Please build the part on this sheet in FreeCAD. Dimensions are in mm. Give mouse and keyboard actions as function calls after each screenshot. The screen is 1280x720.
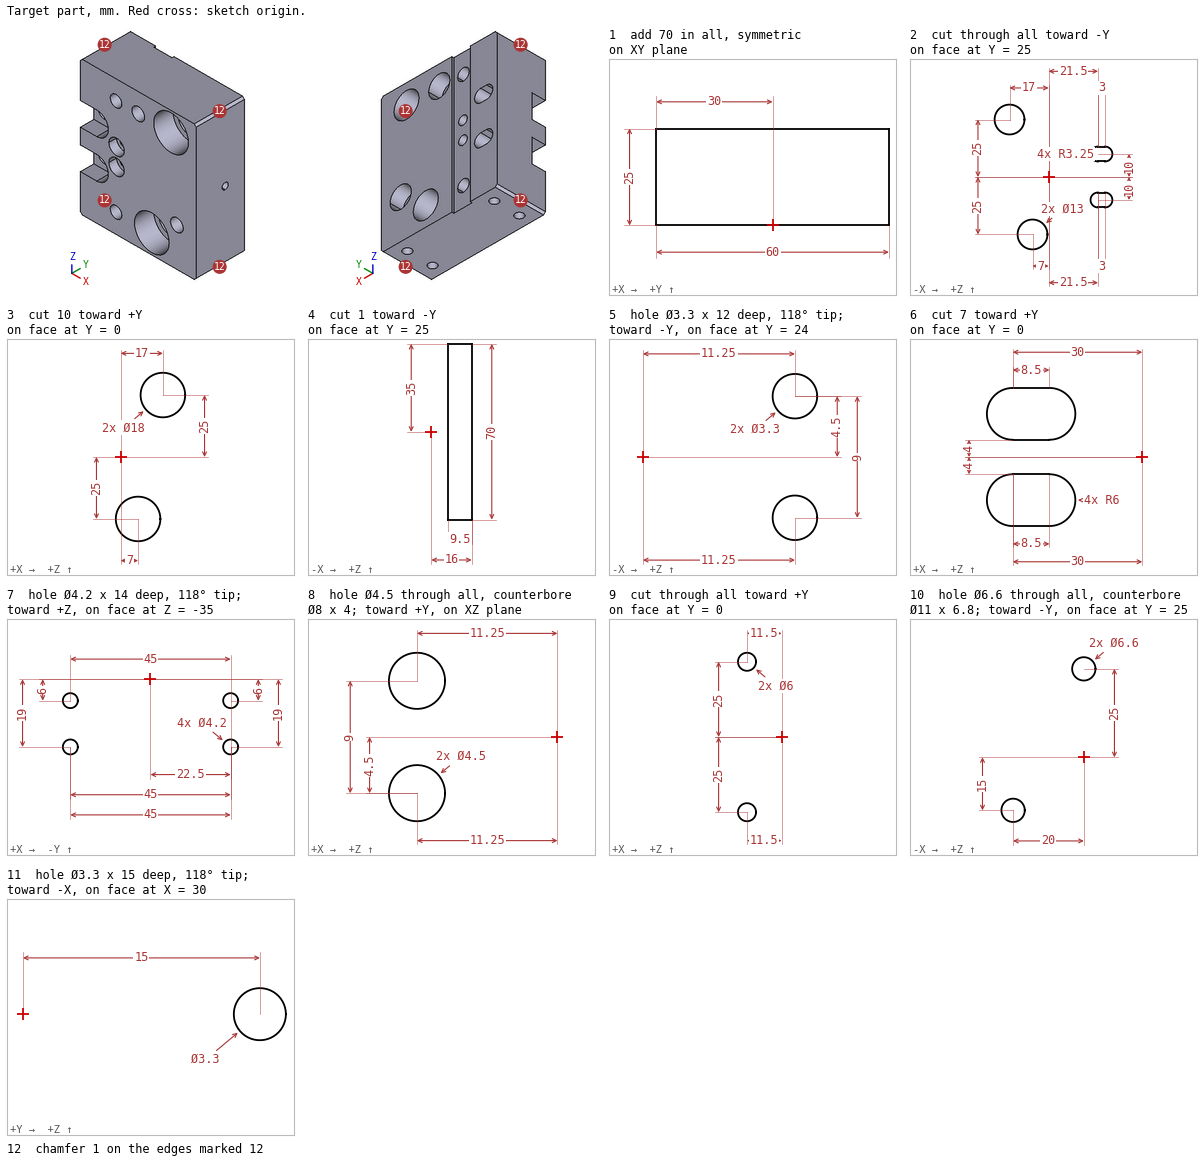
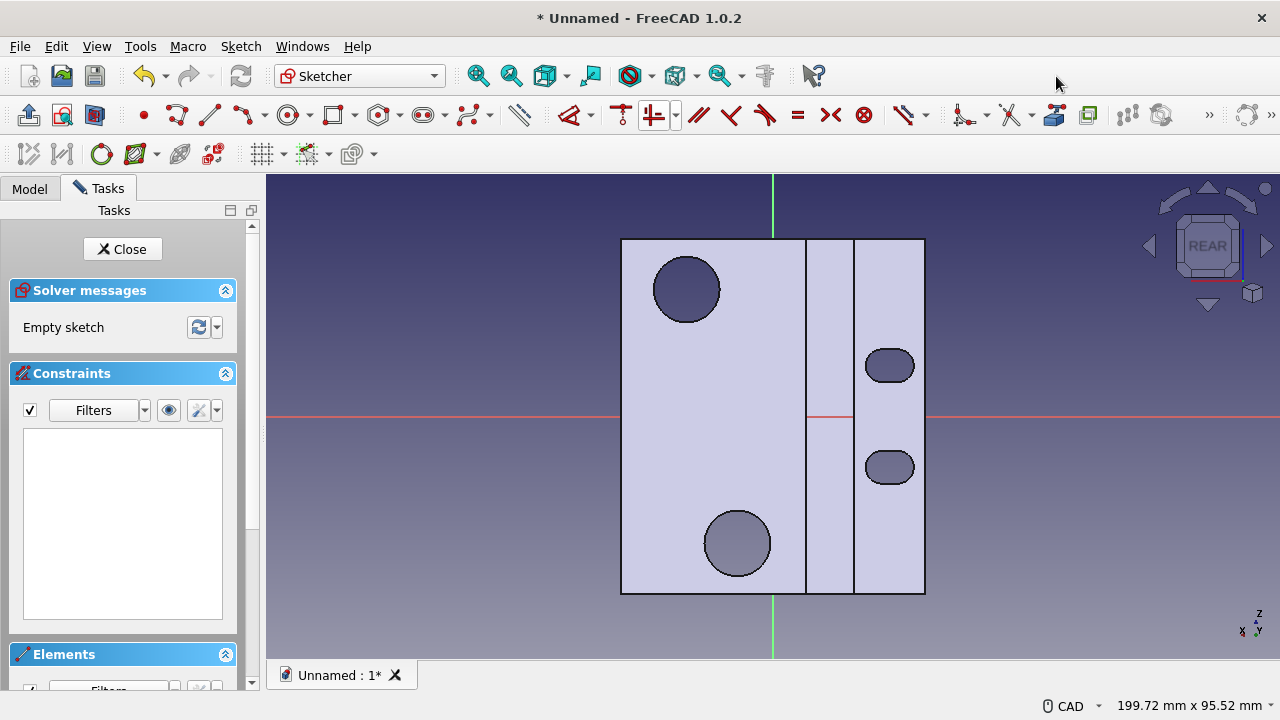
click(95, 116)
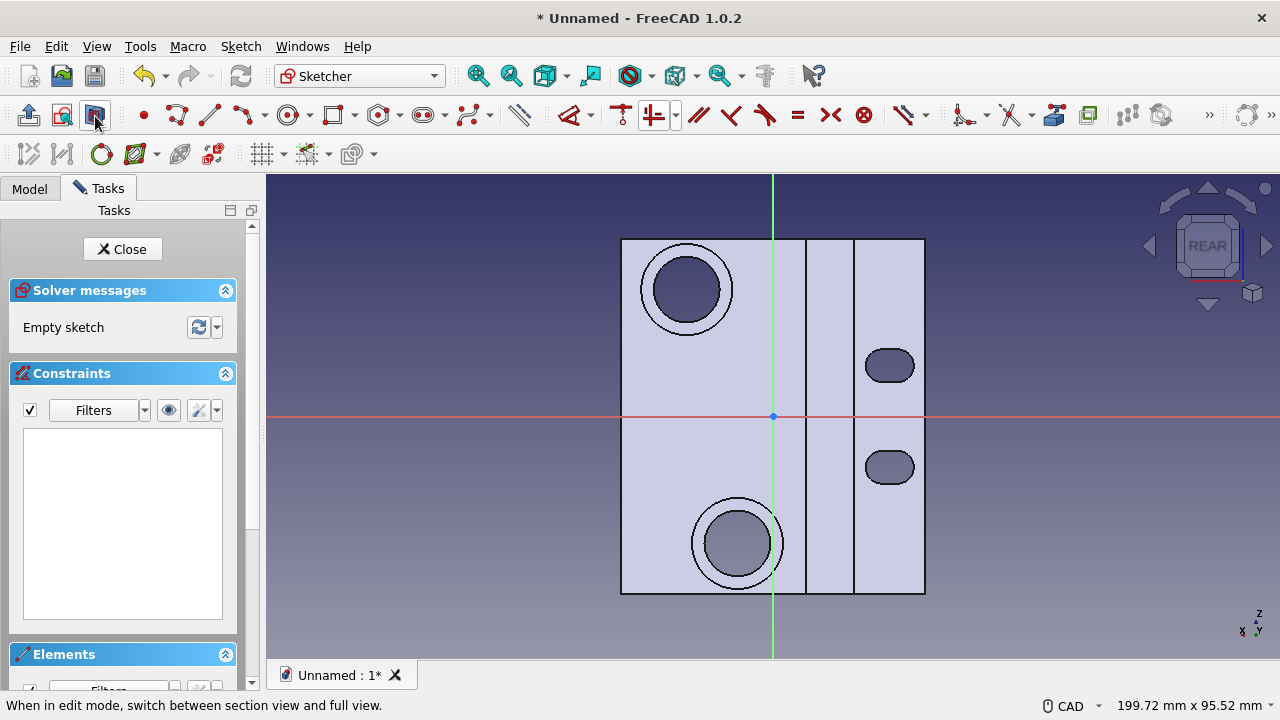
scroll(831, 417, up, 8)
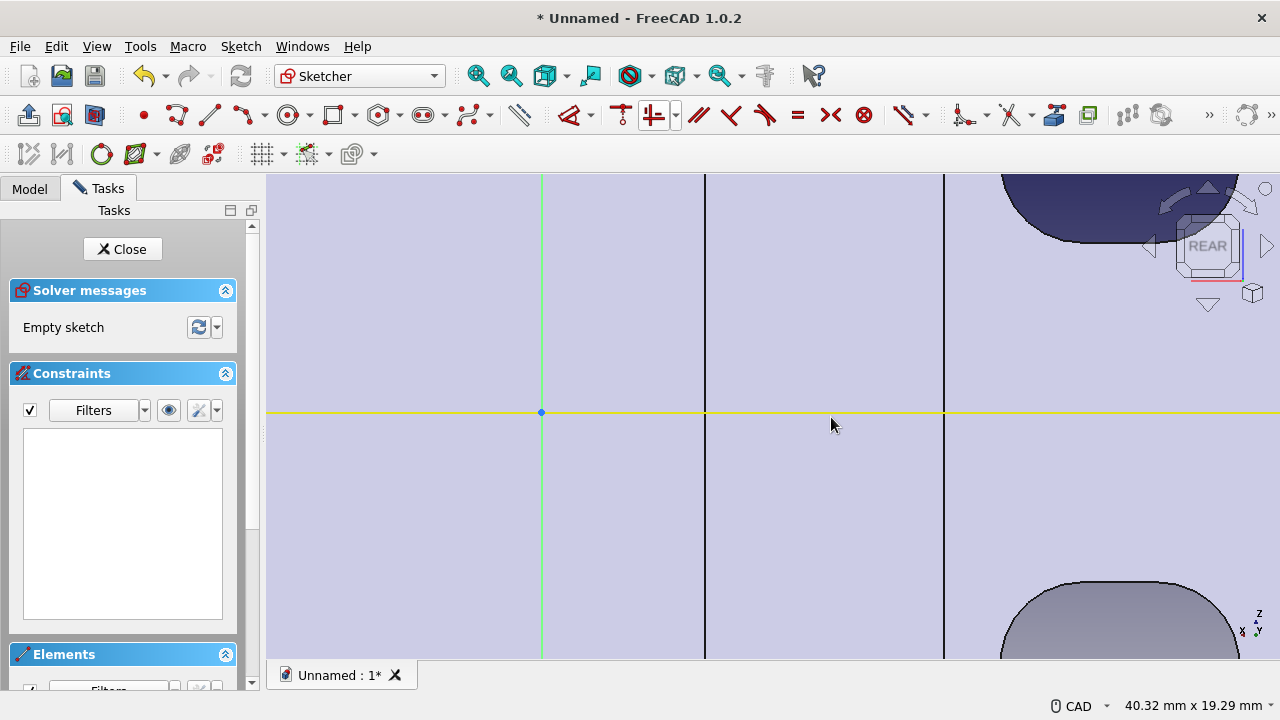
key(g)
key(c)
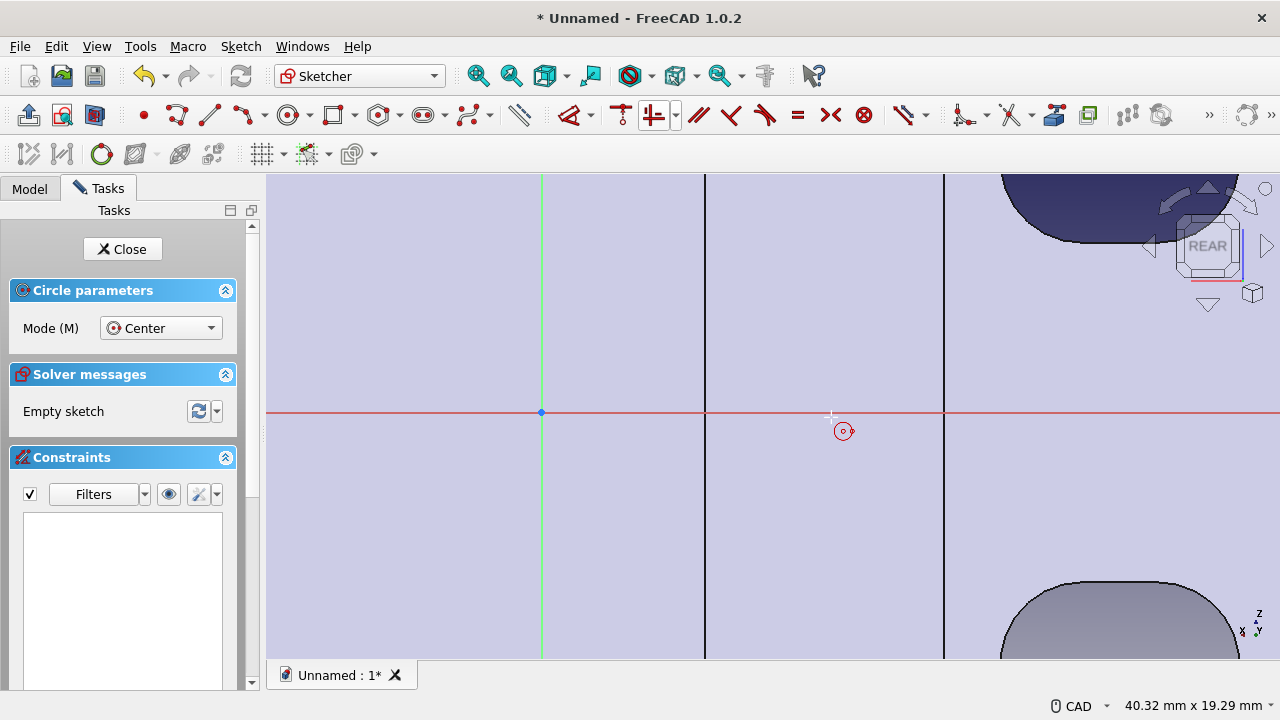
click(824, 299)
move(854, 270)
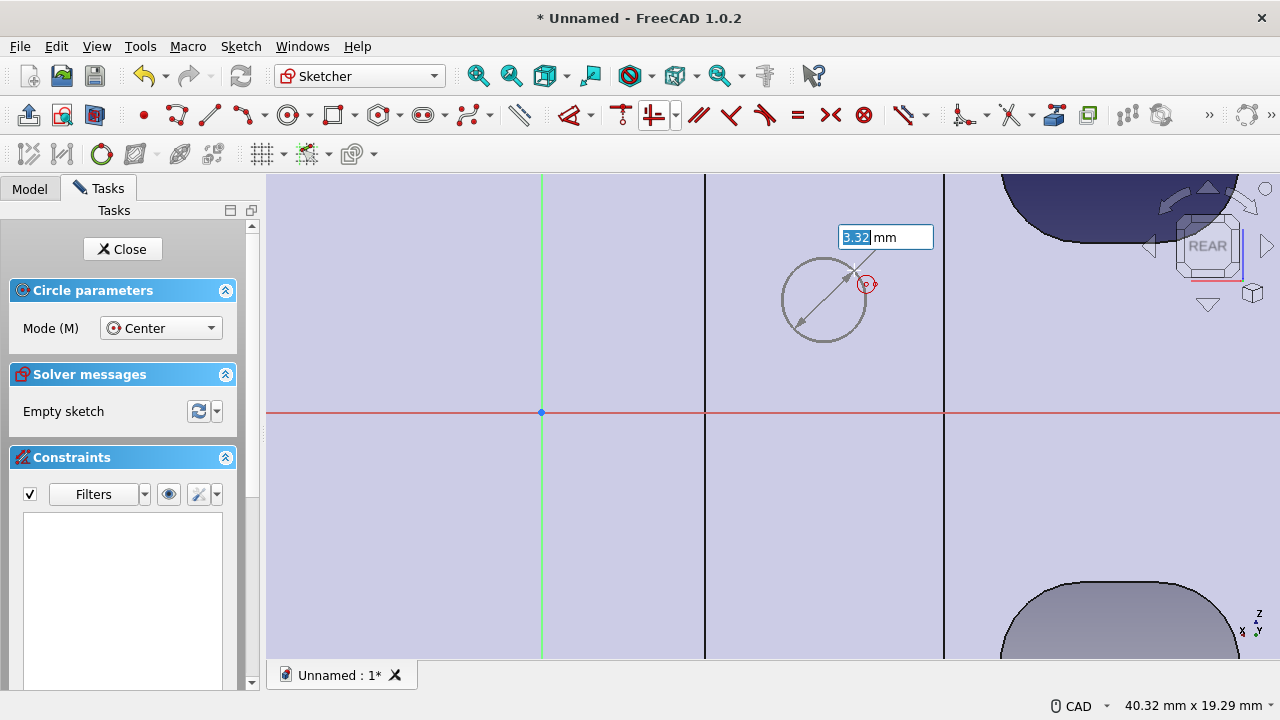
text(3.3)
key(Return)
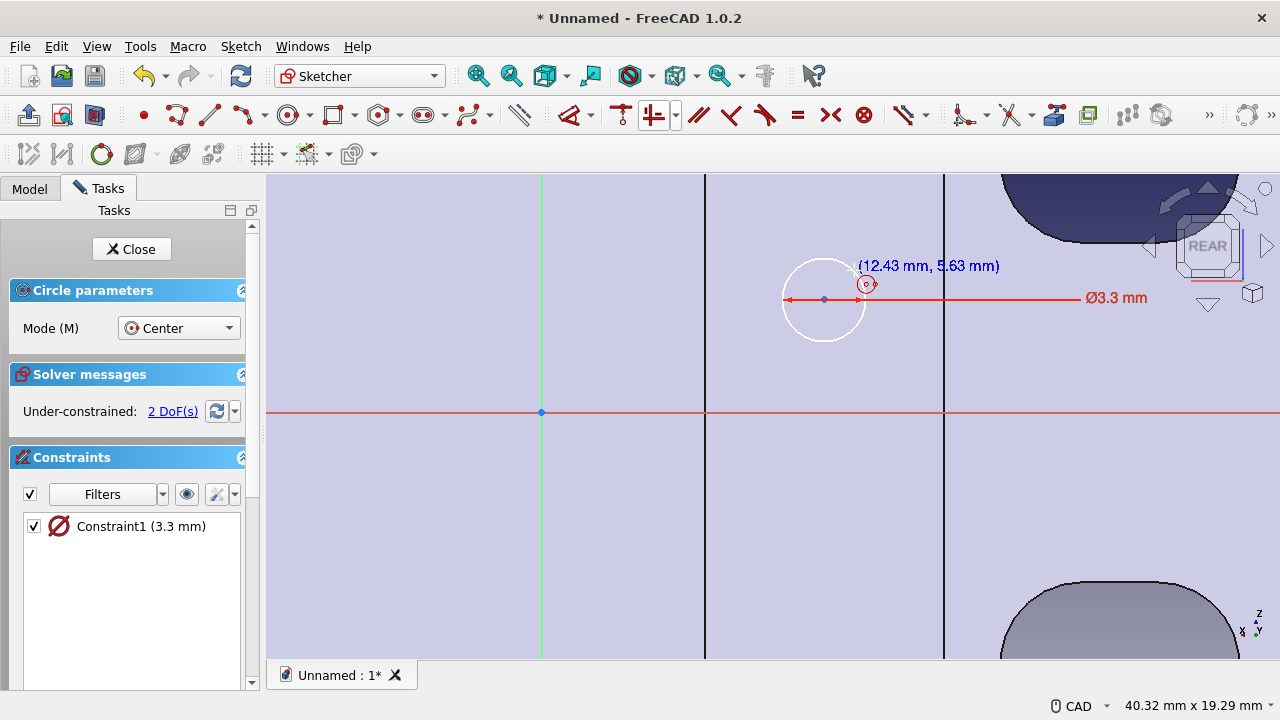
click(824, 526)
move(854, 496)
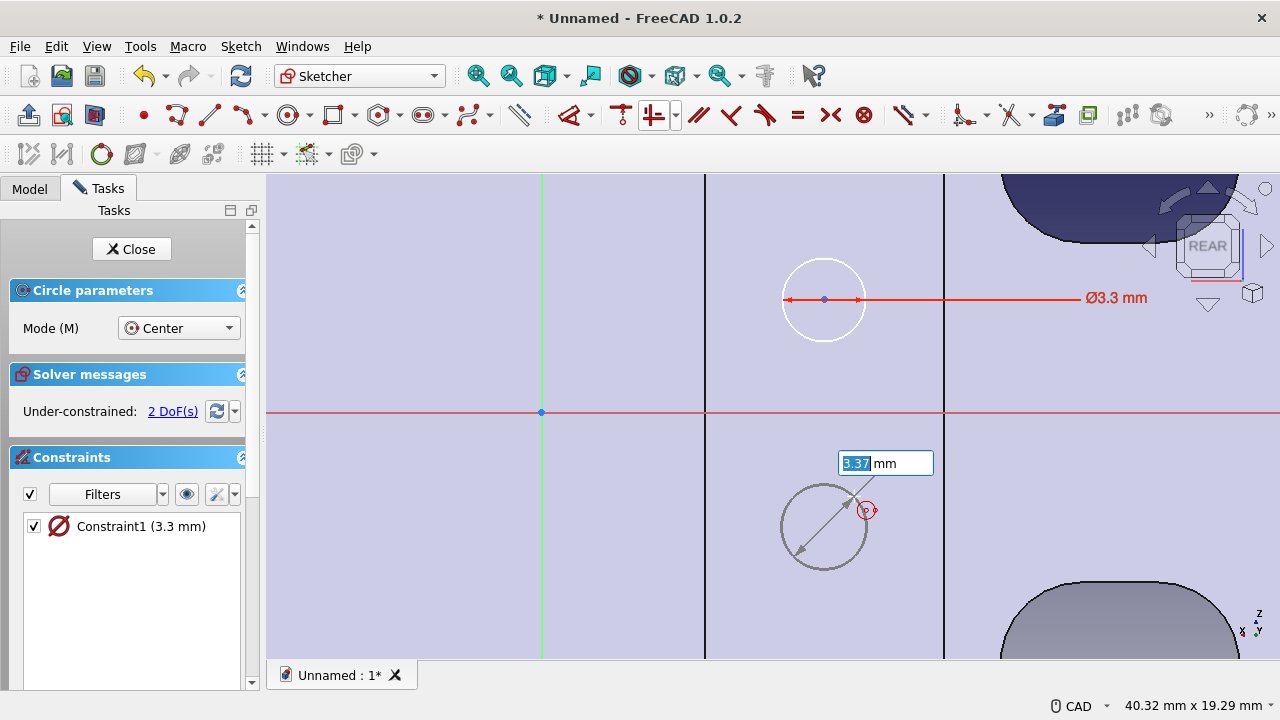
text(3.3)
key(Return)
key(Escape)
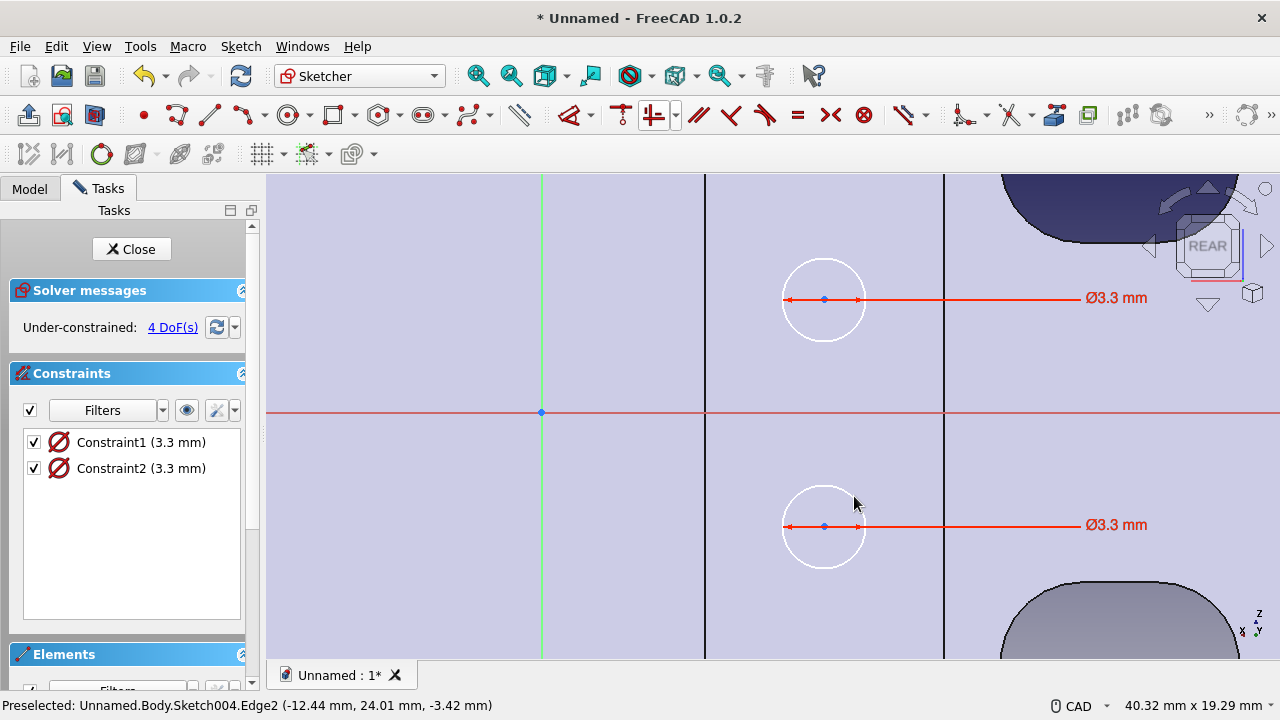
key(d)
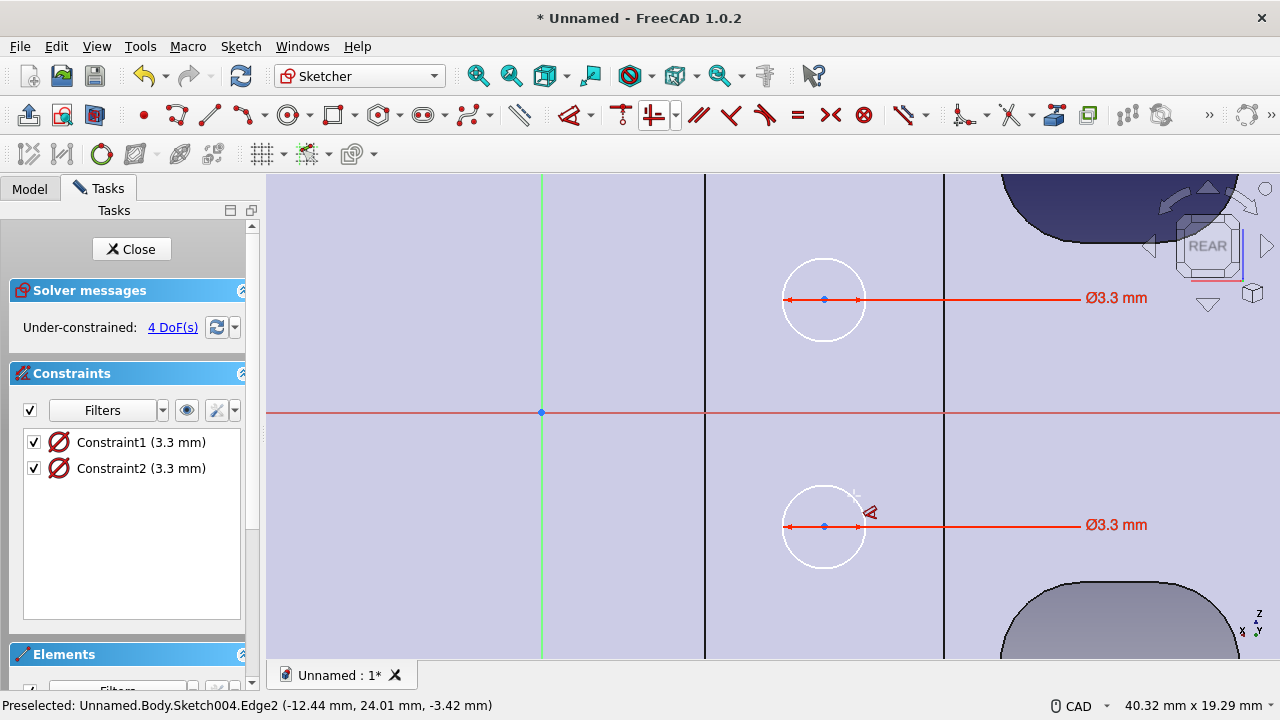
click(824, 300)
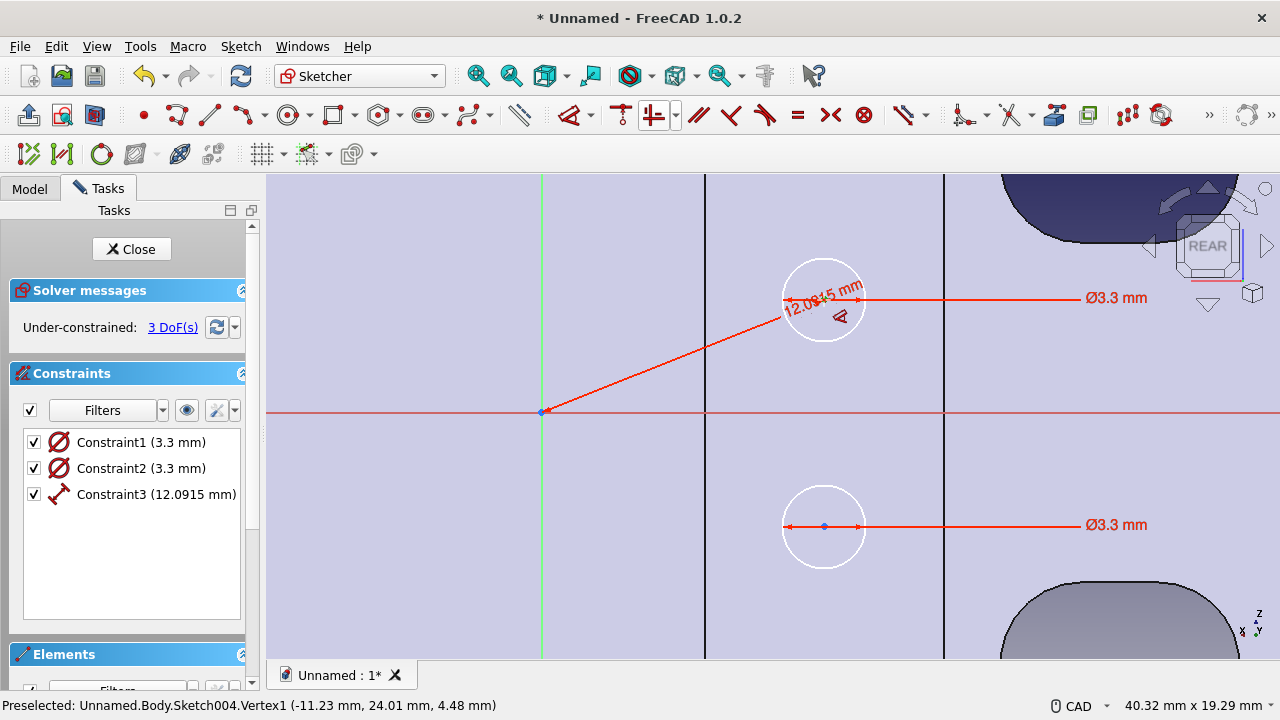
click(824, 527)
click(858, 361)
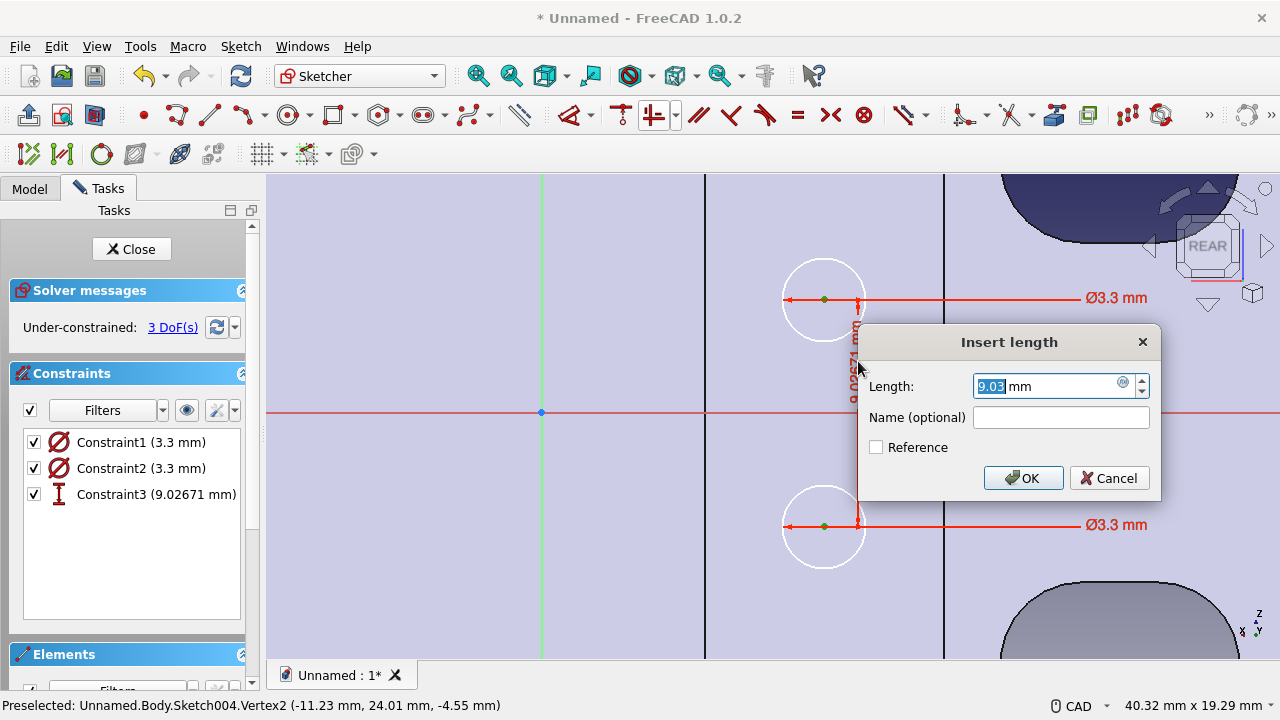
text(9)
key(Return)